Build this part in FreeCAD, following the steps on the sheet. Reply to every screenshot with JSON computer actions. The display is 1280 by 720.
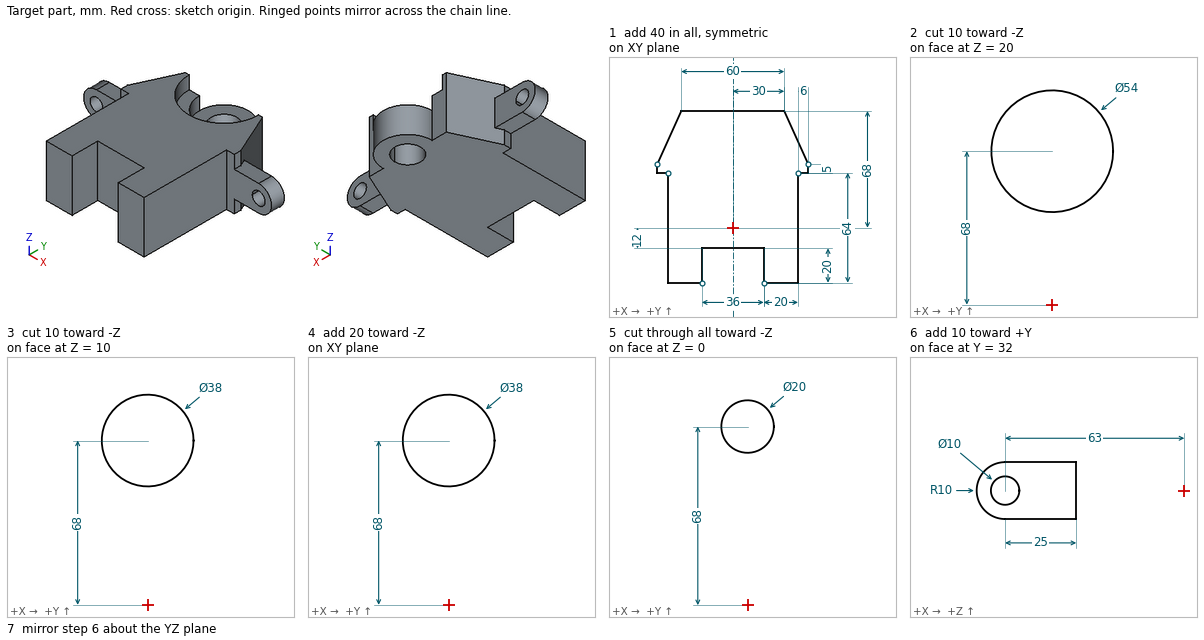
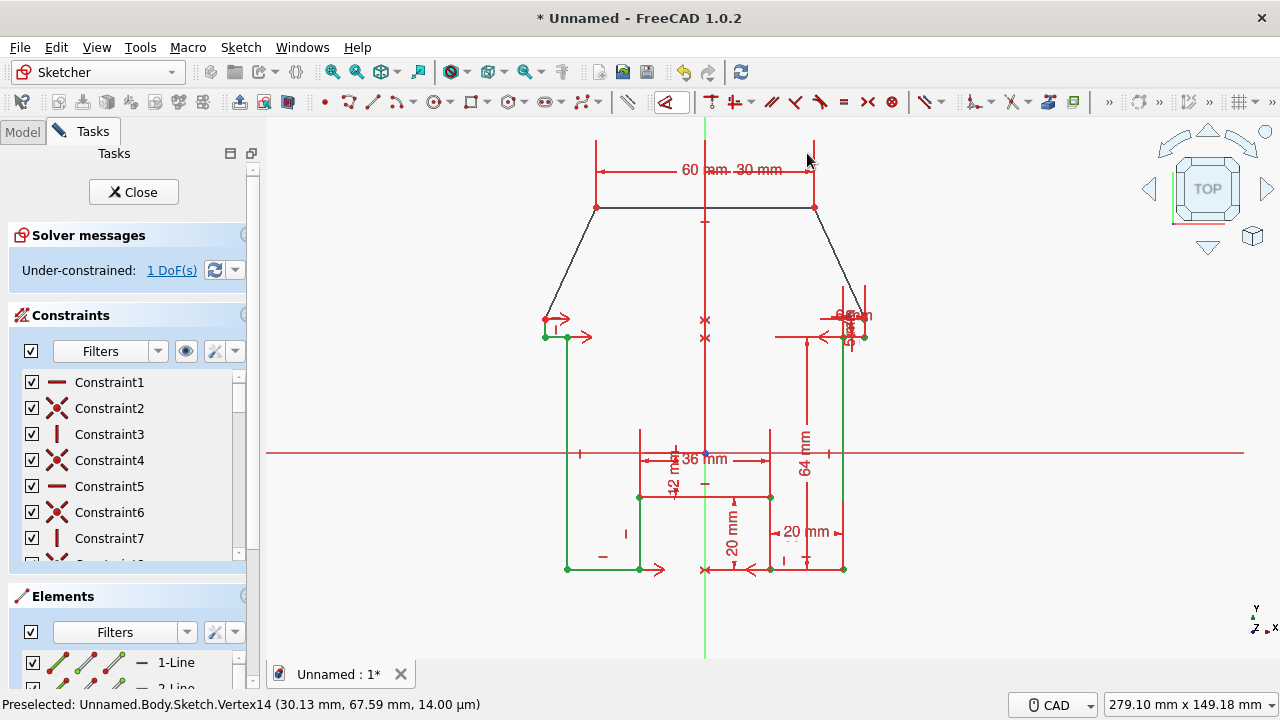
{"action": "left_click", "coordinate": [814, 208]}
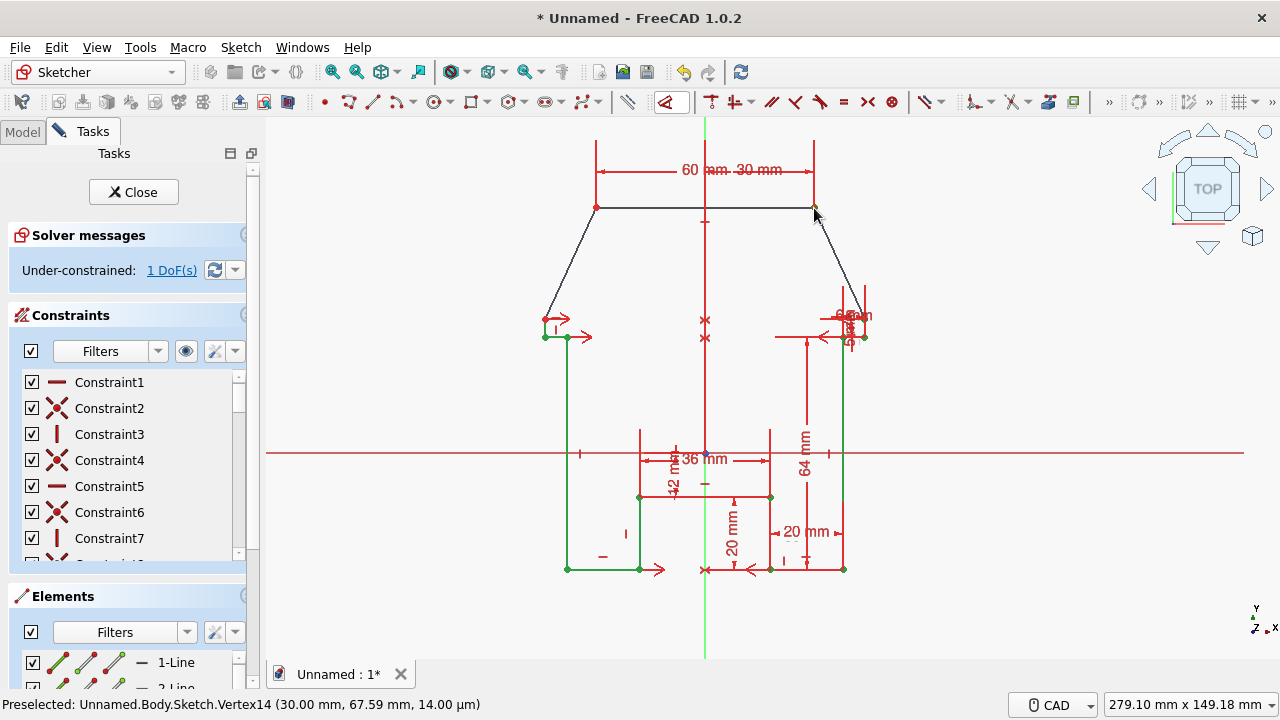
{"action": "key", "text": "i"}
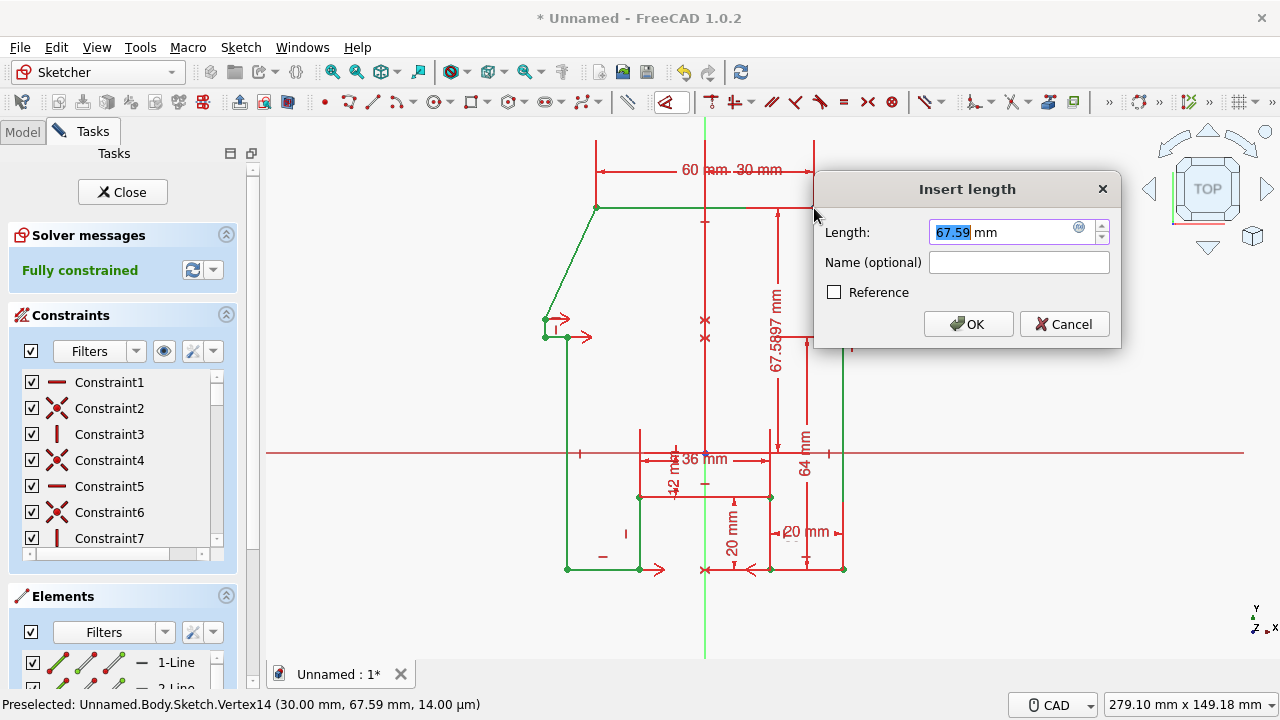
{"action": "type", "text": "68"}
{"action": "key", "text": "Return"}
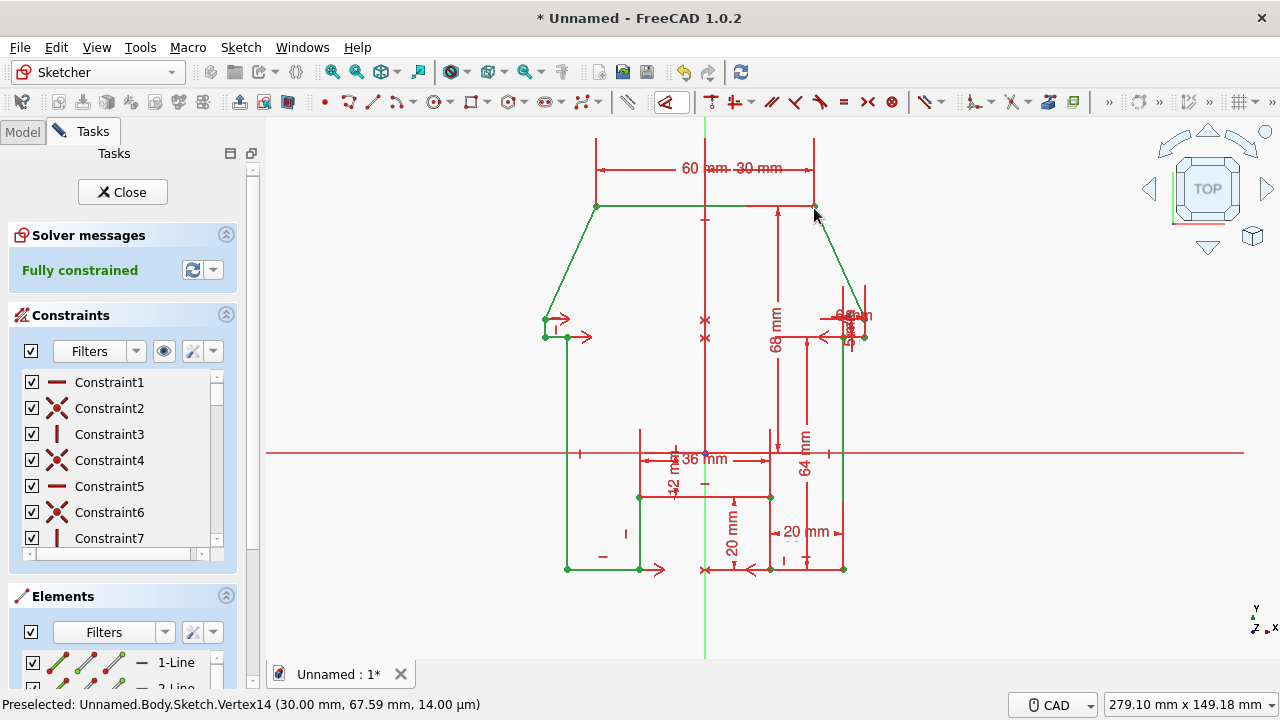
{"action": "left_click", "coordinate": [123, 192]}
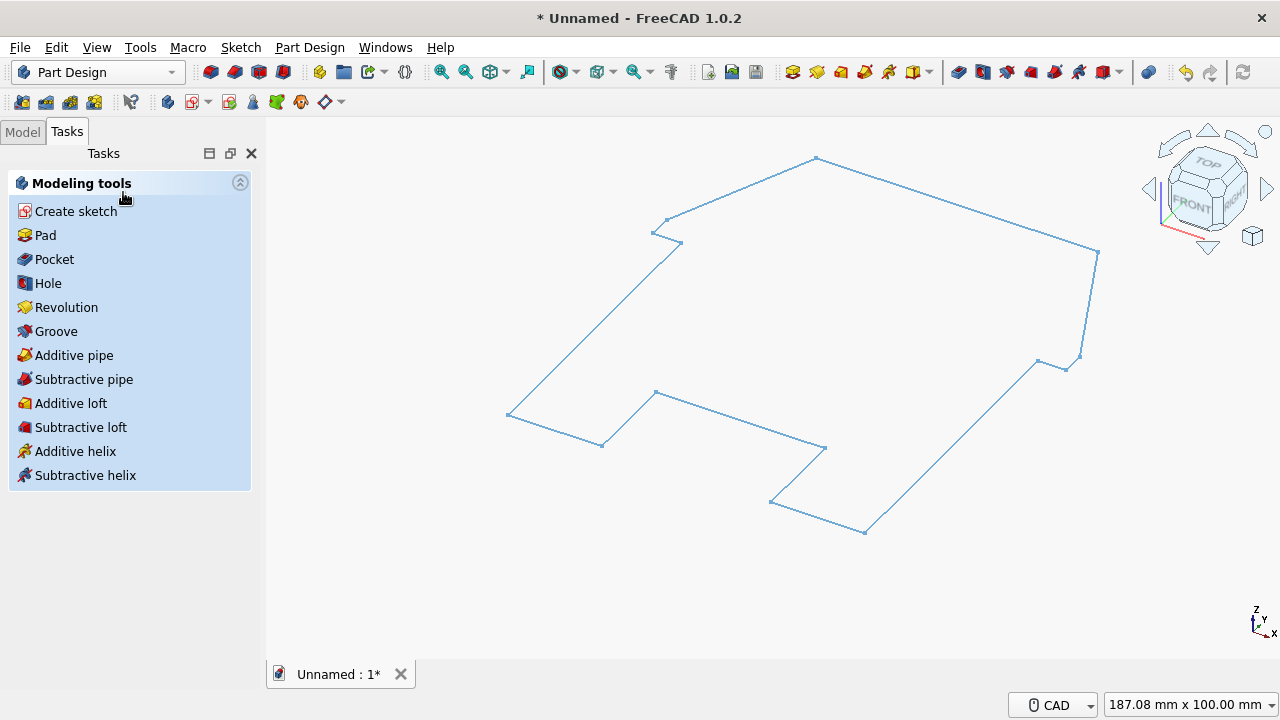
{"action": "left_click", "coordinate": [794, 72]}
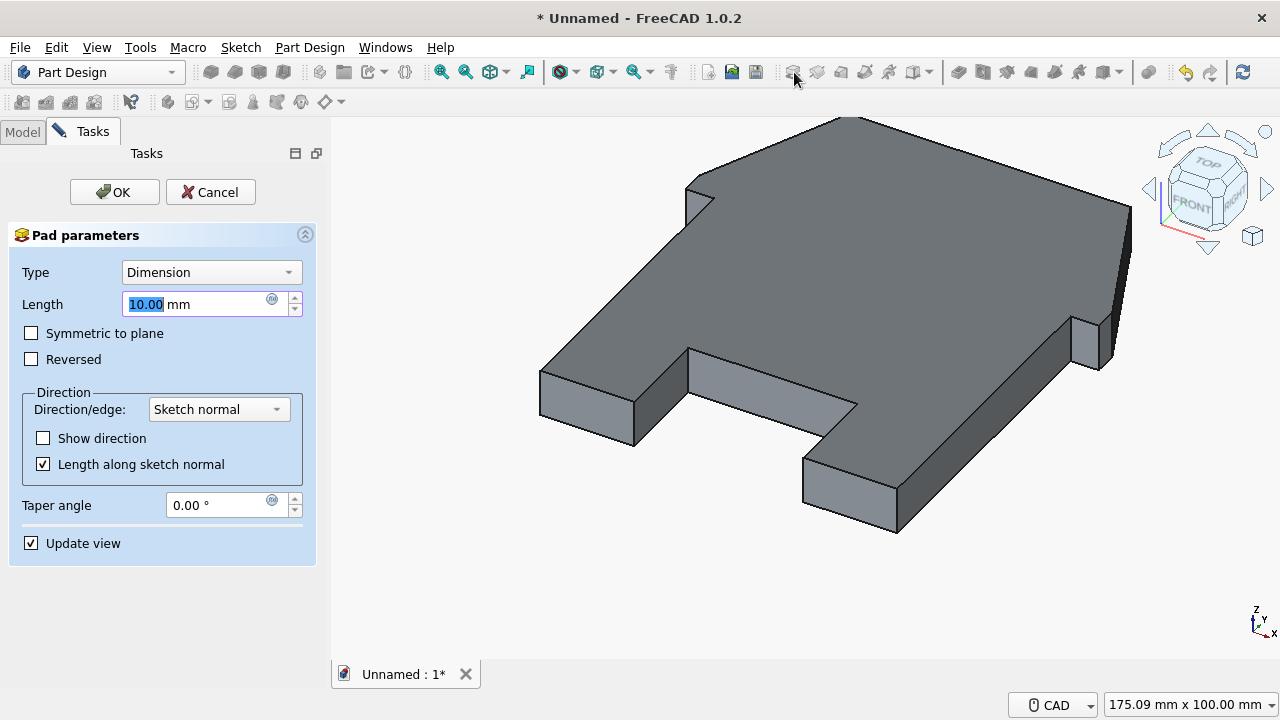
{"action": "type", "text": "40"}
{"action": "key", "text": "Tab"}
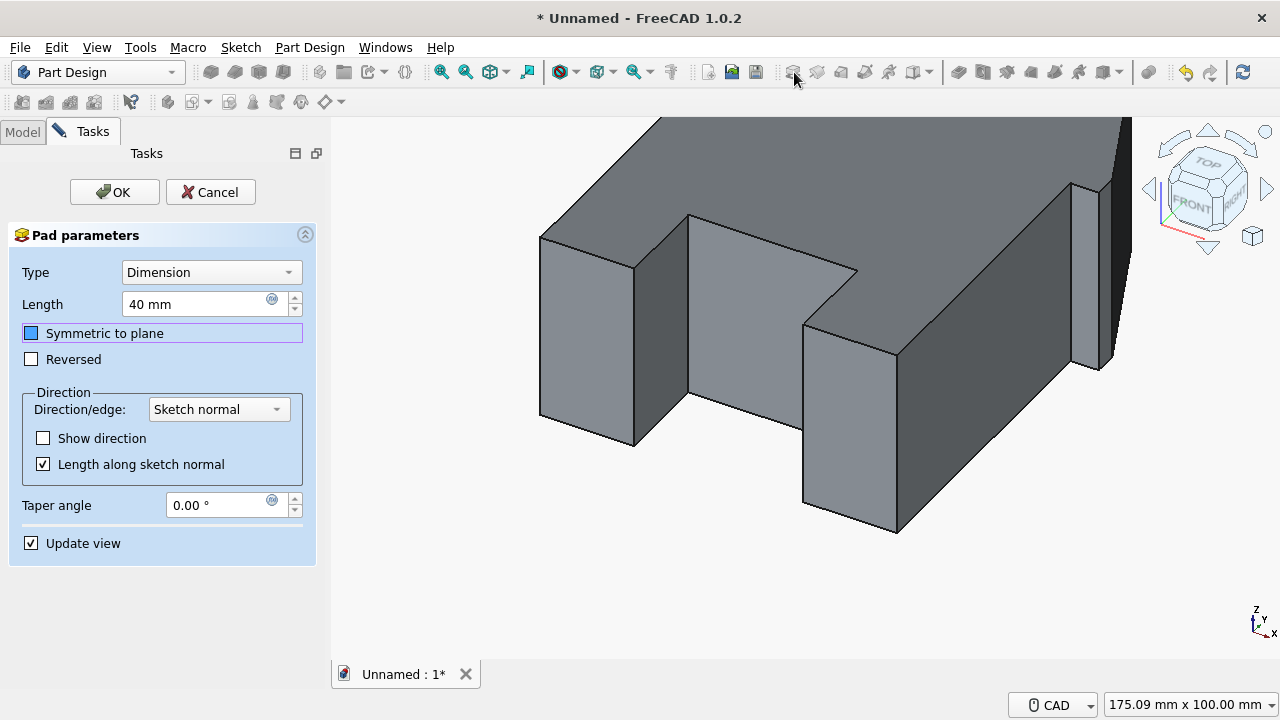
{"action": "left_click", "coordinate": [30, 333]}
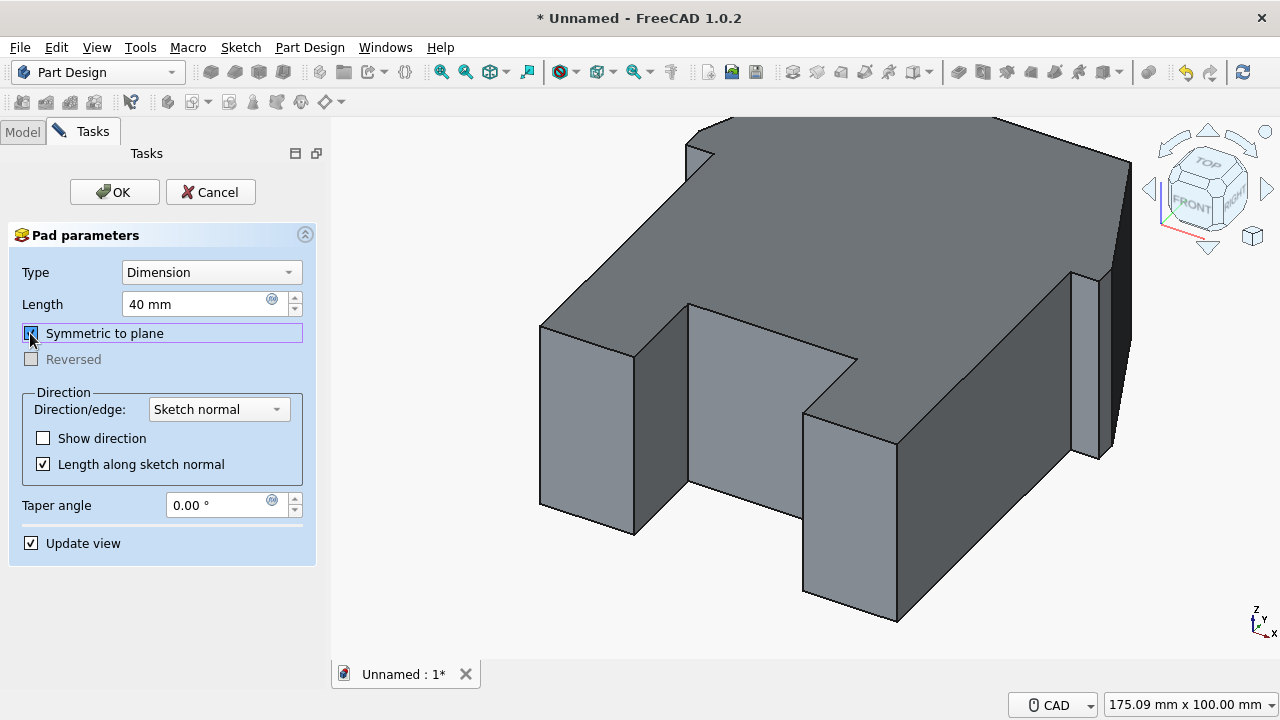
{"action": "left_click", "coordinate": [115, 192]}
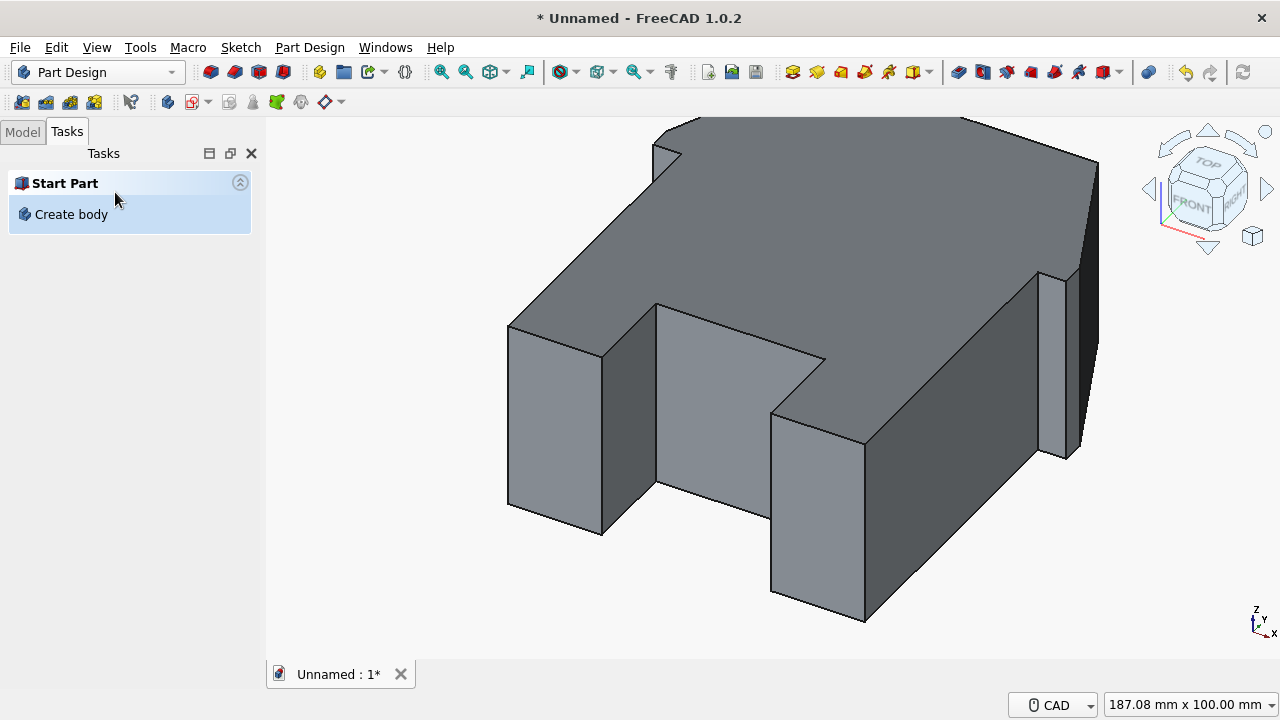
{"action": "left_click", "coordinate": [442, 72]}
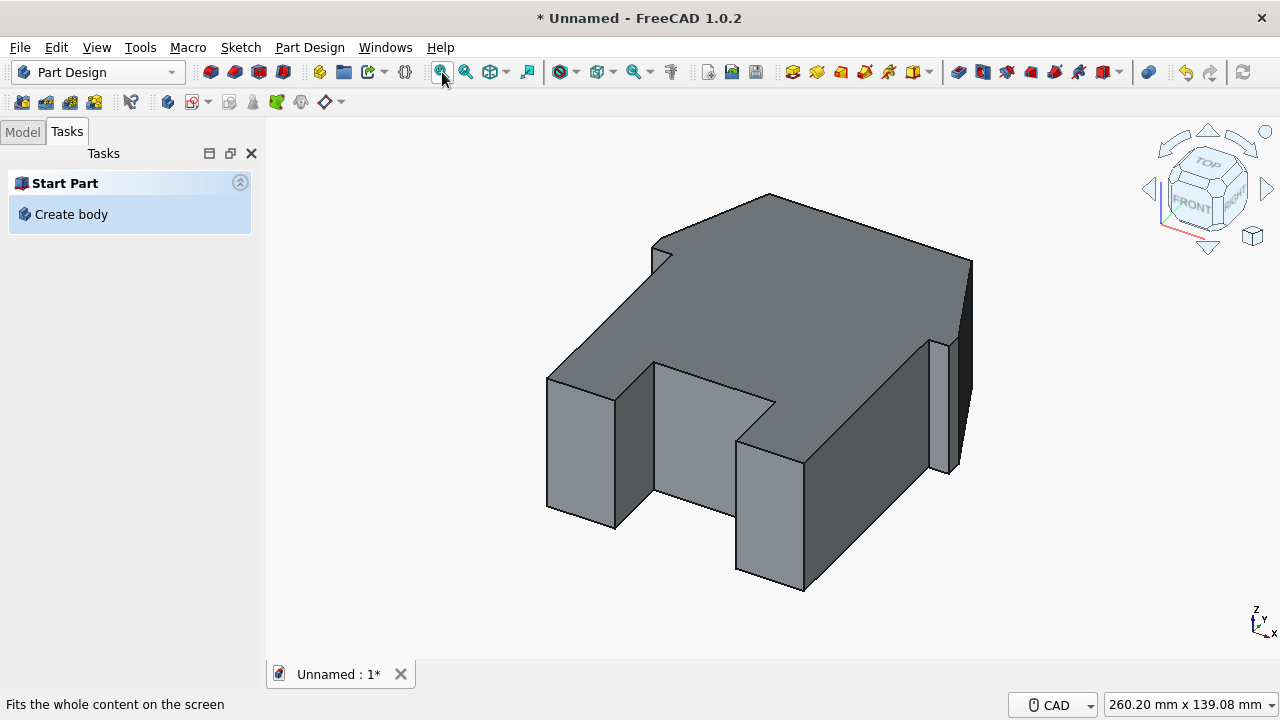
{"action": "left_click", "coordinate": [801, 296]}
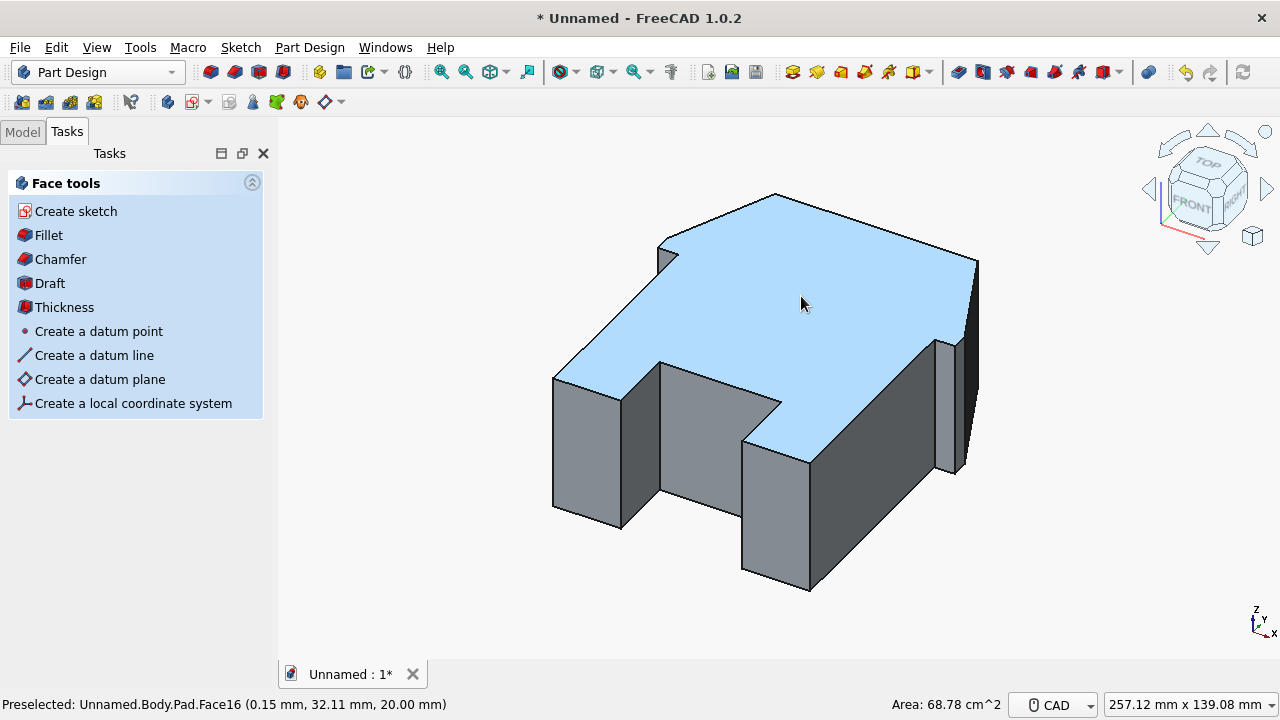
{"action": "left_click", "coordinate": [192, 102]}